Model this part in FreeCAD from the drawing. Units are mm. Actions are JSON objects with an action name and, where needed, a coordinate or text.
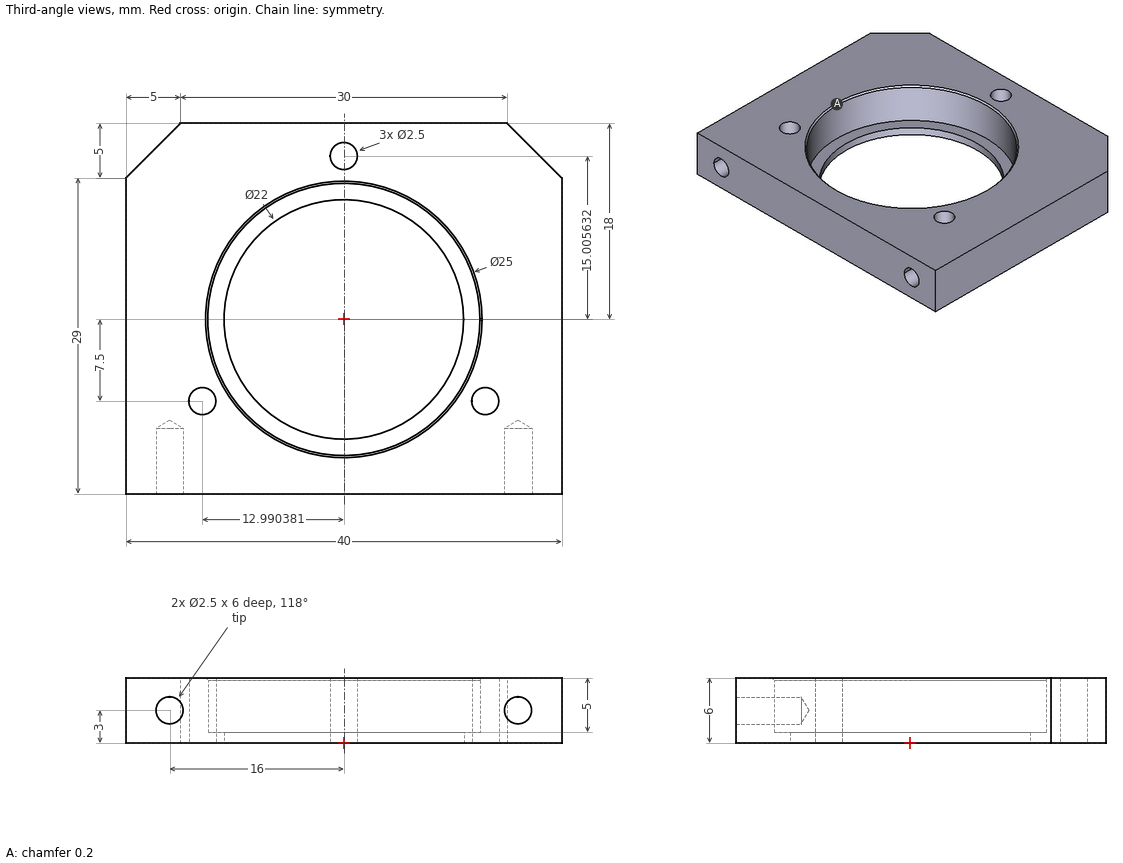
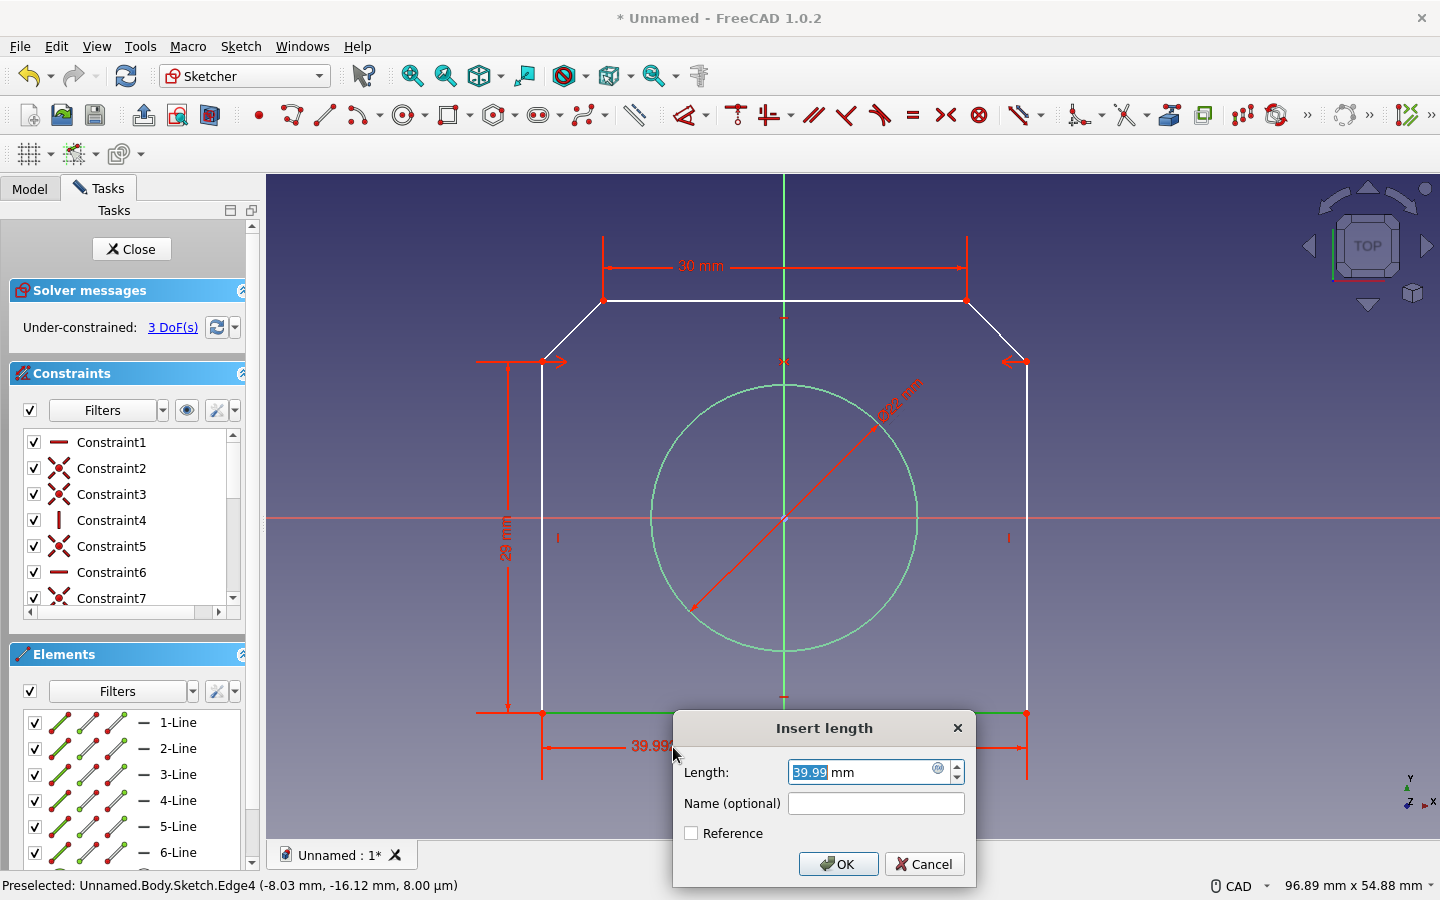
{"action": "type", "text": "40"}
{"action": "key", "text": "Return"}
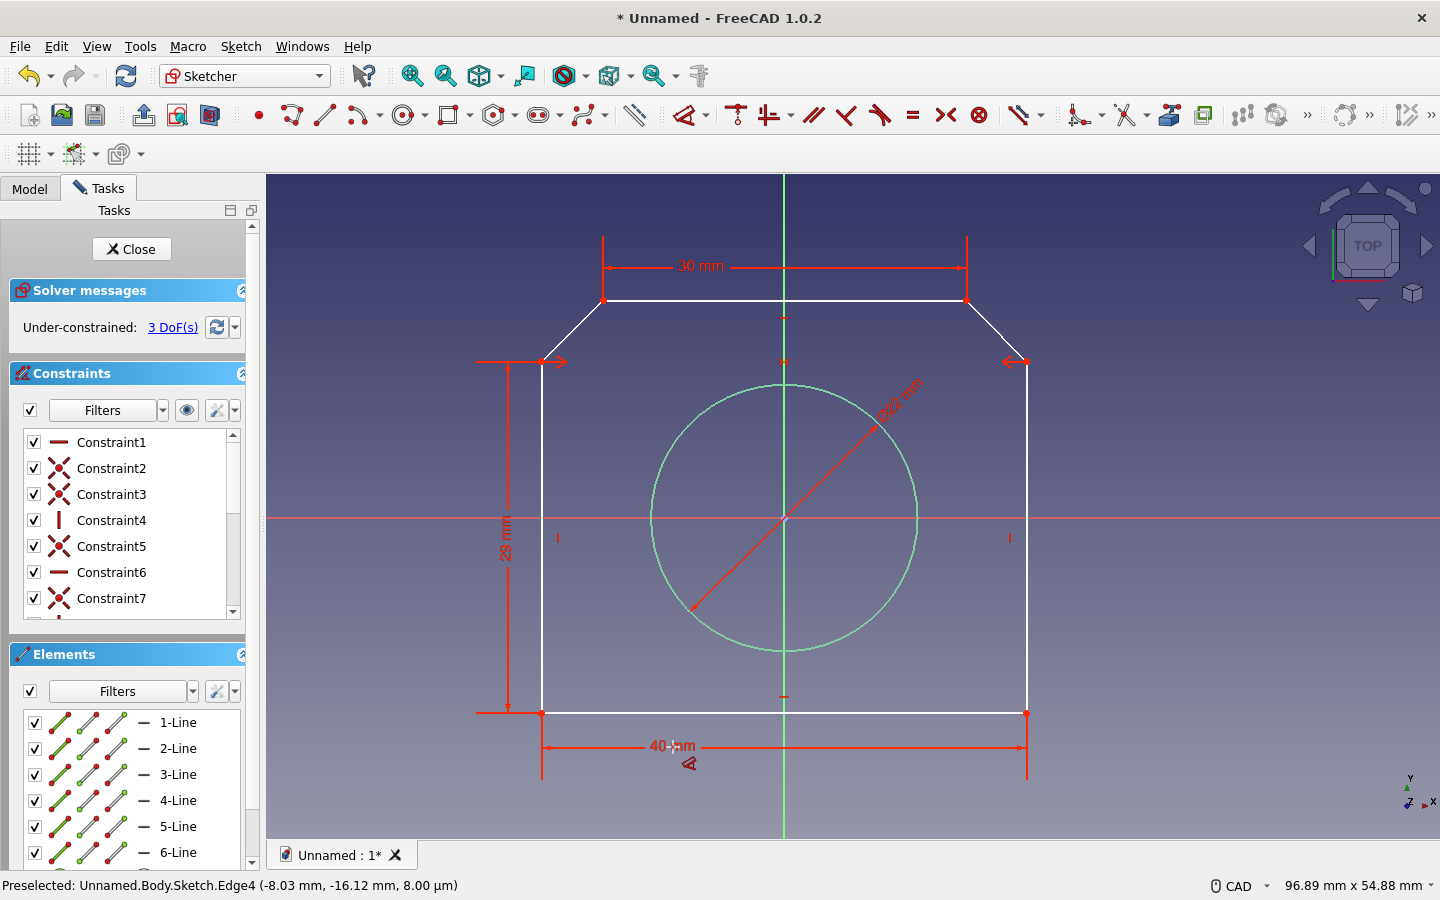
{"action": "left_click", "coordinate": [585, 319]}
{"action": "left_click", "coordinate": [572, 267]}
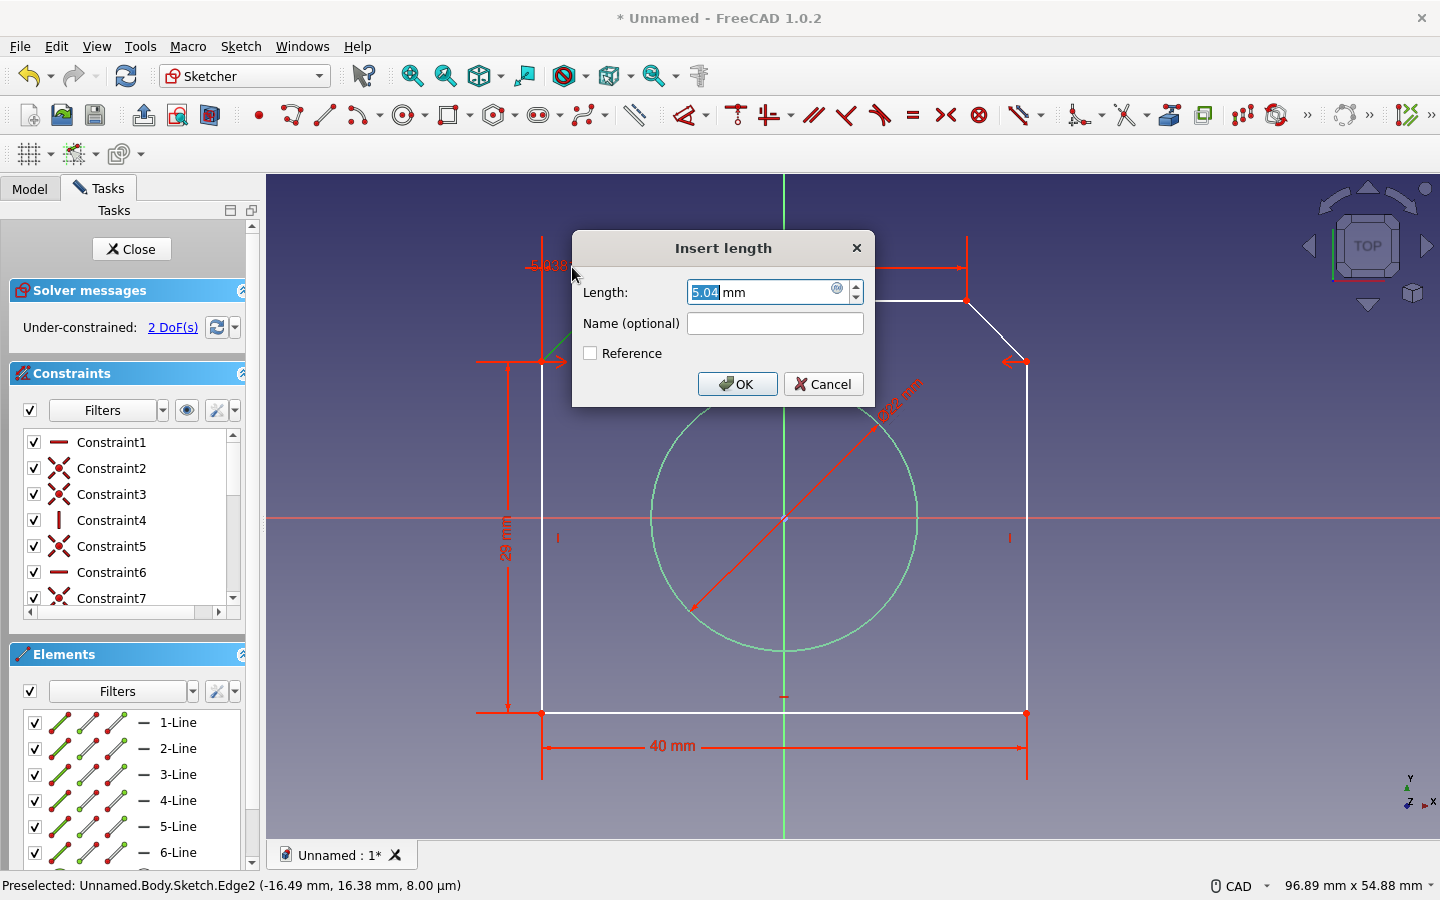
{"action": "type", "text": "5"}
{"action": "key", "text": "Return"}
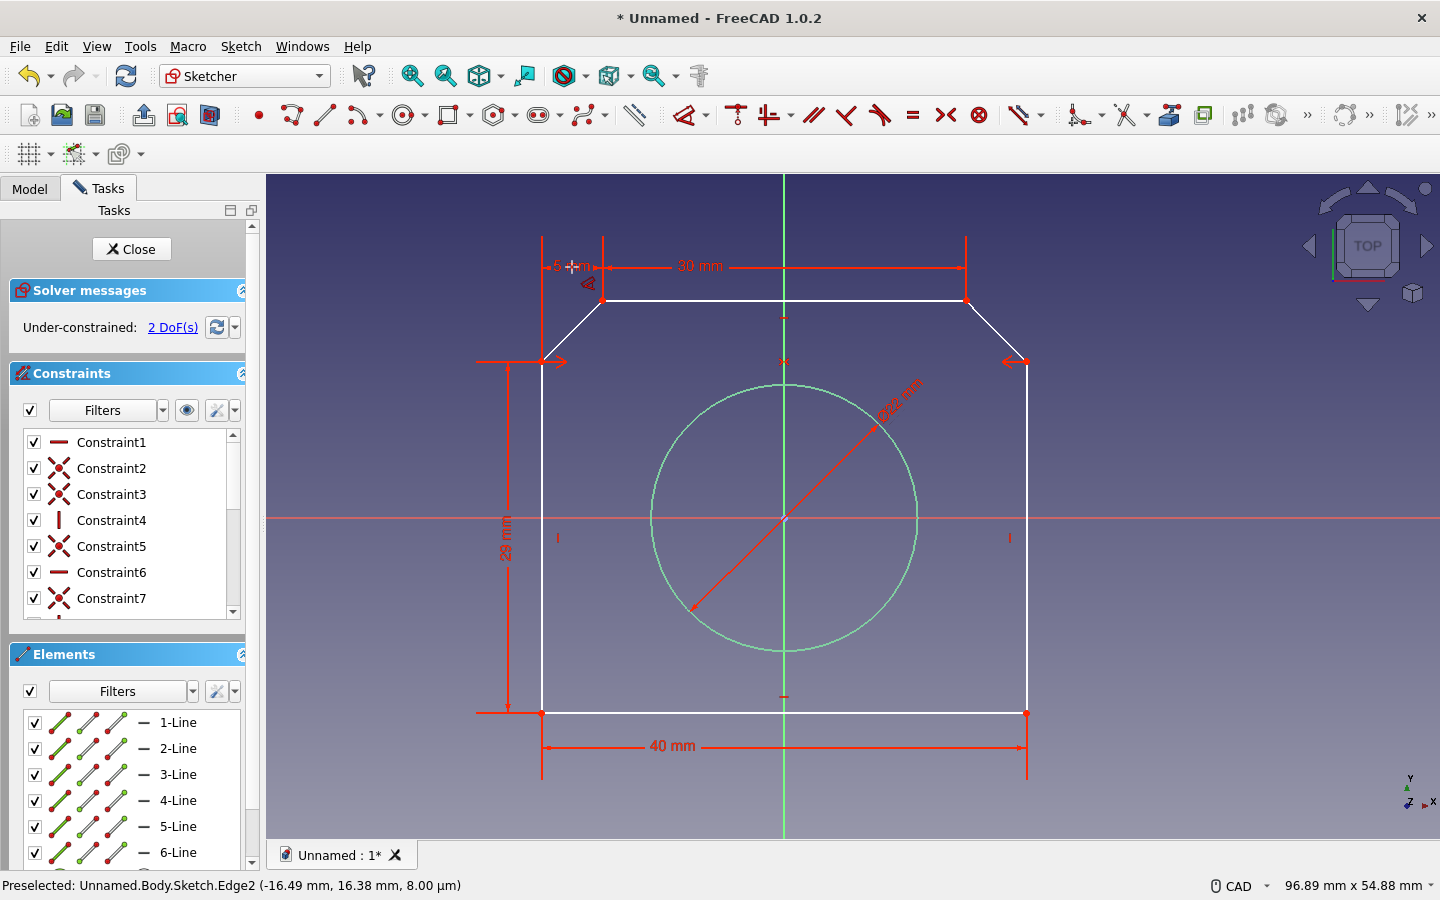
{"action": "left_click", "coordinate": [584, 319]}
{"action": "left_click", "coordinate": [508, 331]}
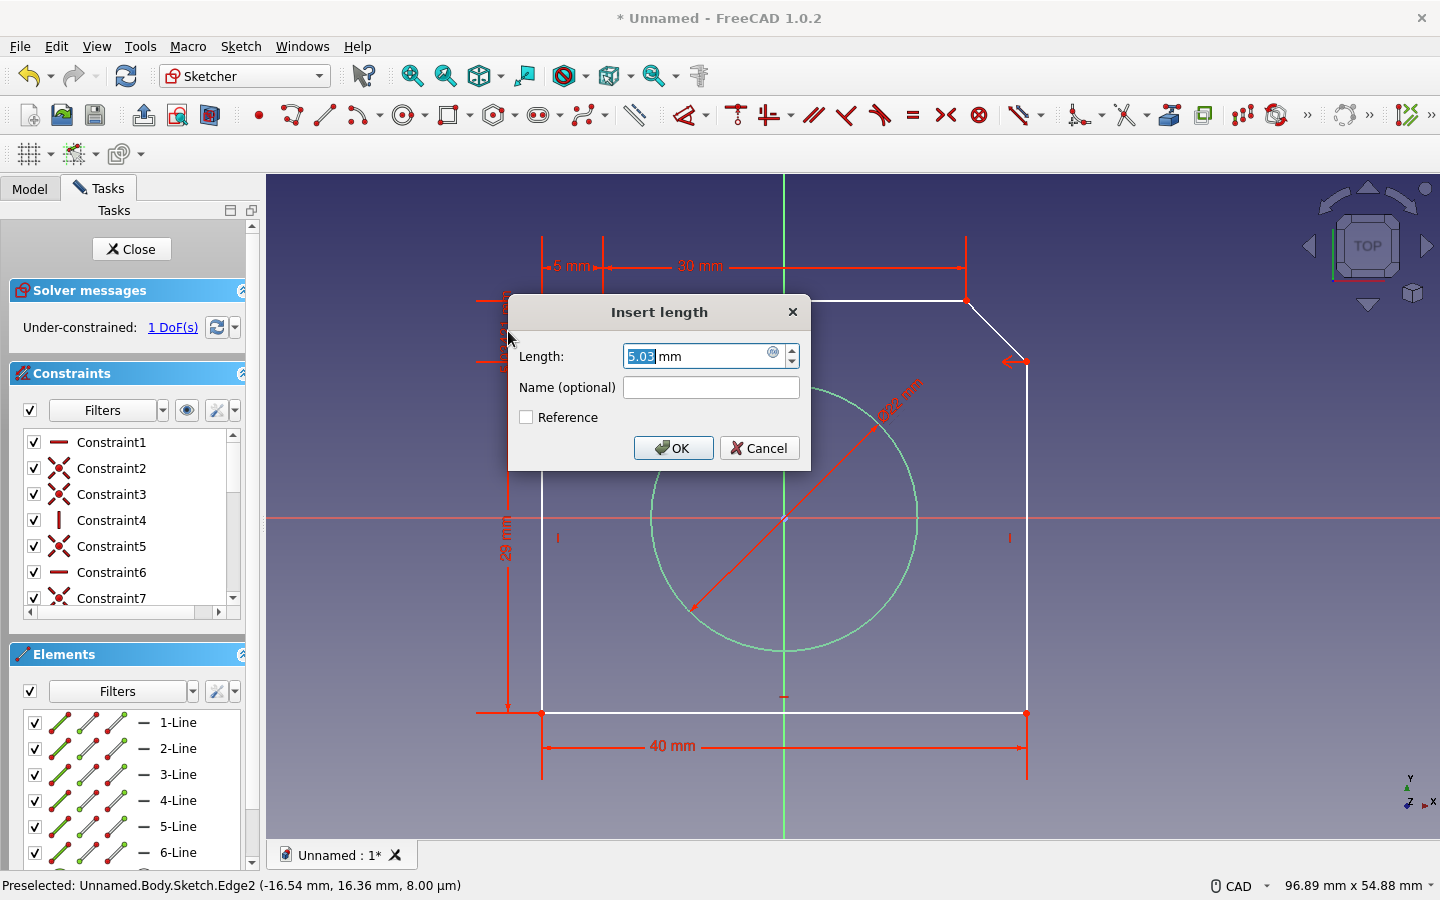
{"action": "type", "text": "5"}
{"action": "key", "text": "Return"}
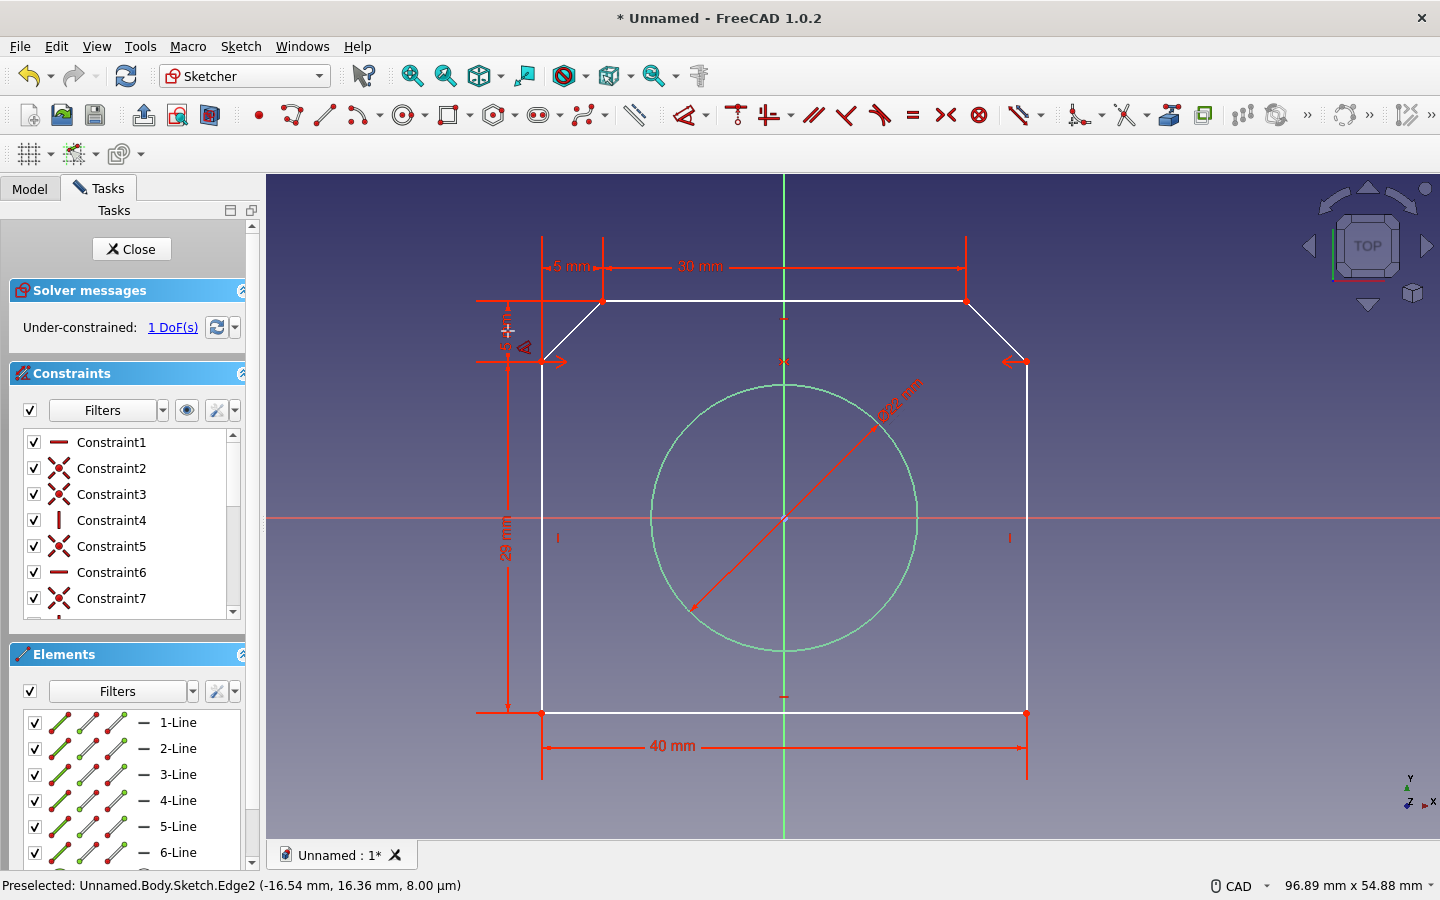
{"action": "left_click", "coordinate": [966, 301]}
{"action": "left_click", "coordinate": [1000, 410]}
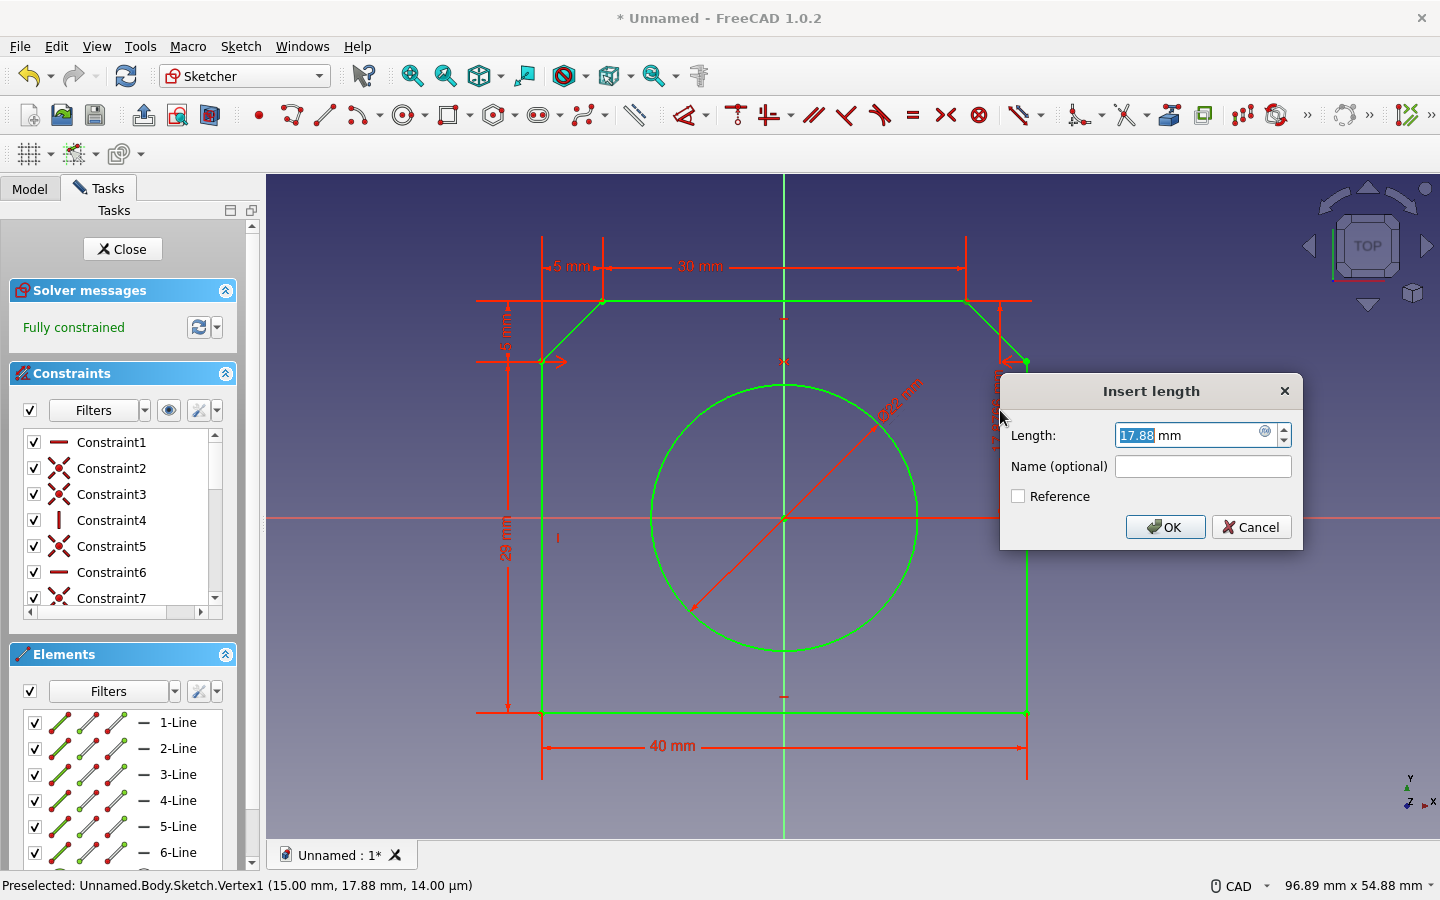
{"action": "type", "text": "18"}
{"action": "key", "text": "Return"}
{"action": "key", "text": "Escape"}